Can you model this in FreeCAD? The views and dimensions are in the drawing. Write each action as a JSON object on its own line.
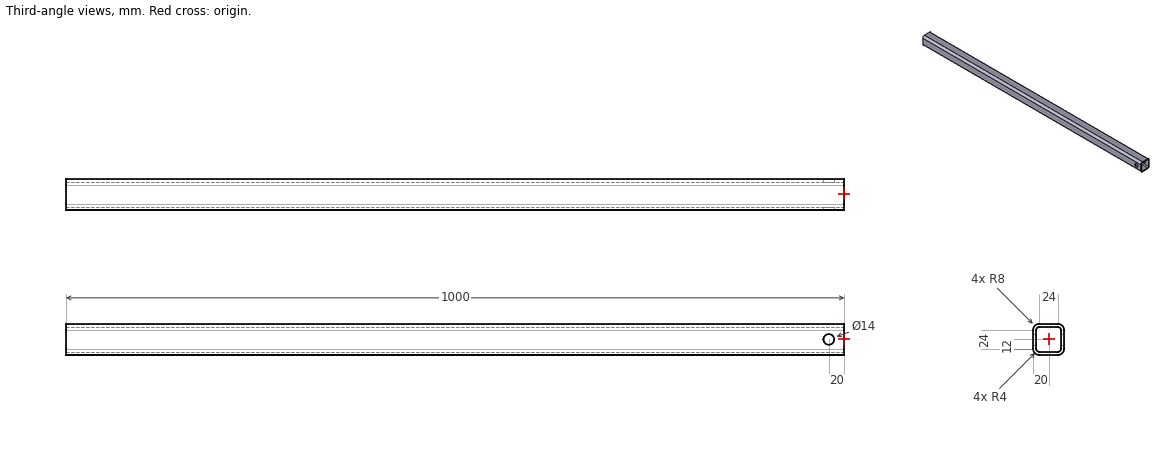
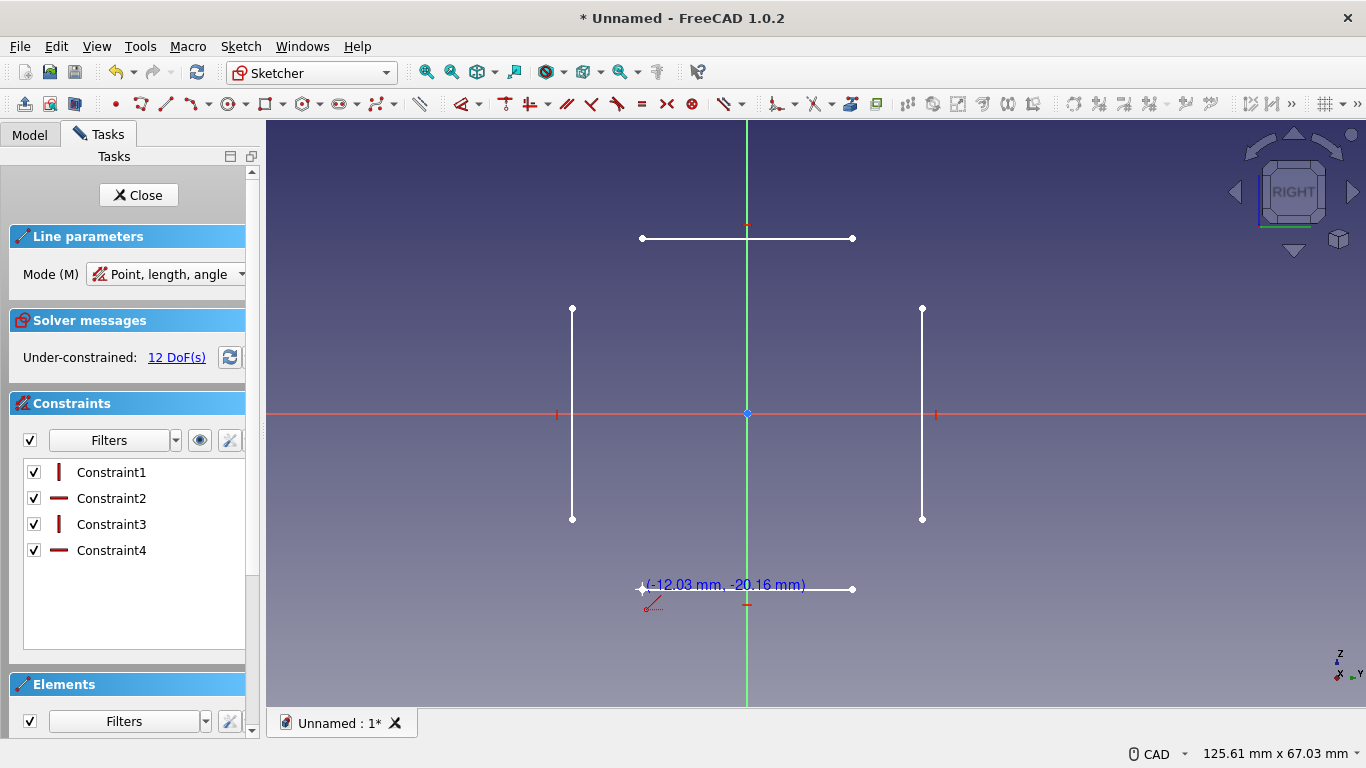
{"action": "left_click", "coordinate": [190, 104]}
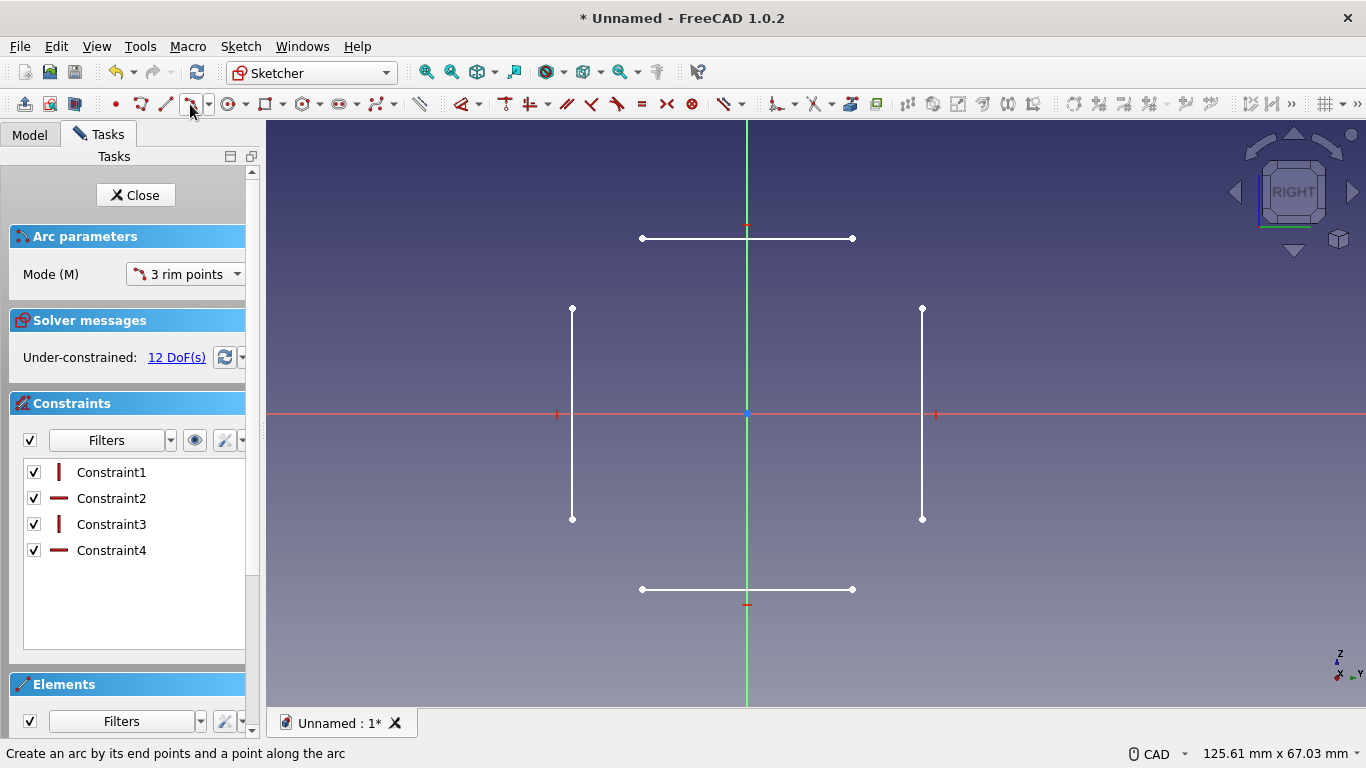
{"action": "left_click", "coordinate": [572, 309]}
{"action": "left_click", "coordinate": [642, 239]}
{"action": "left_click", "coordinate": [593, 259]}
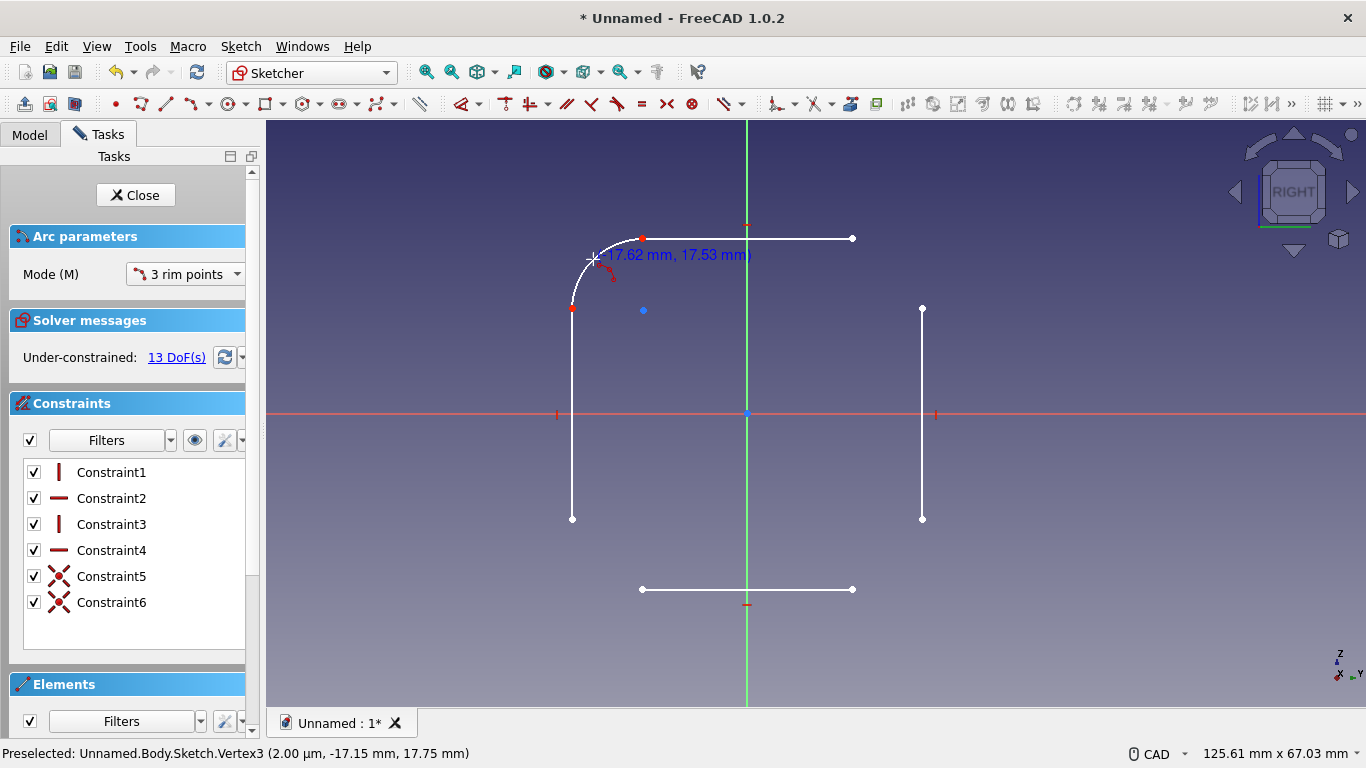
{"action": "left_click", "coordinate": [852, 239]}
{"action": "left_click", "coordinate": [922, 309]}
{"action": "left_click", "coordinate": [902, 259]}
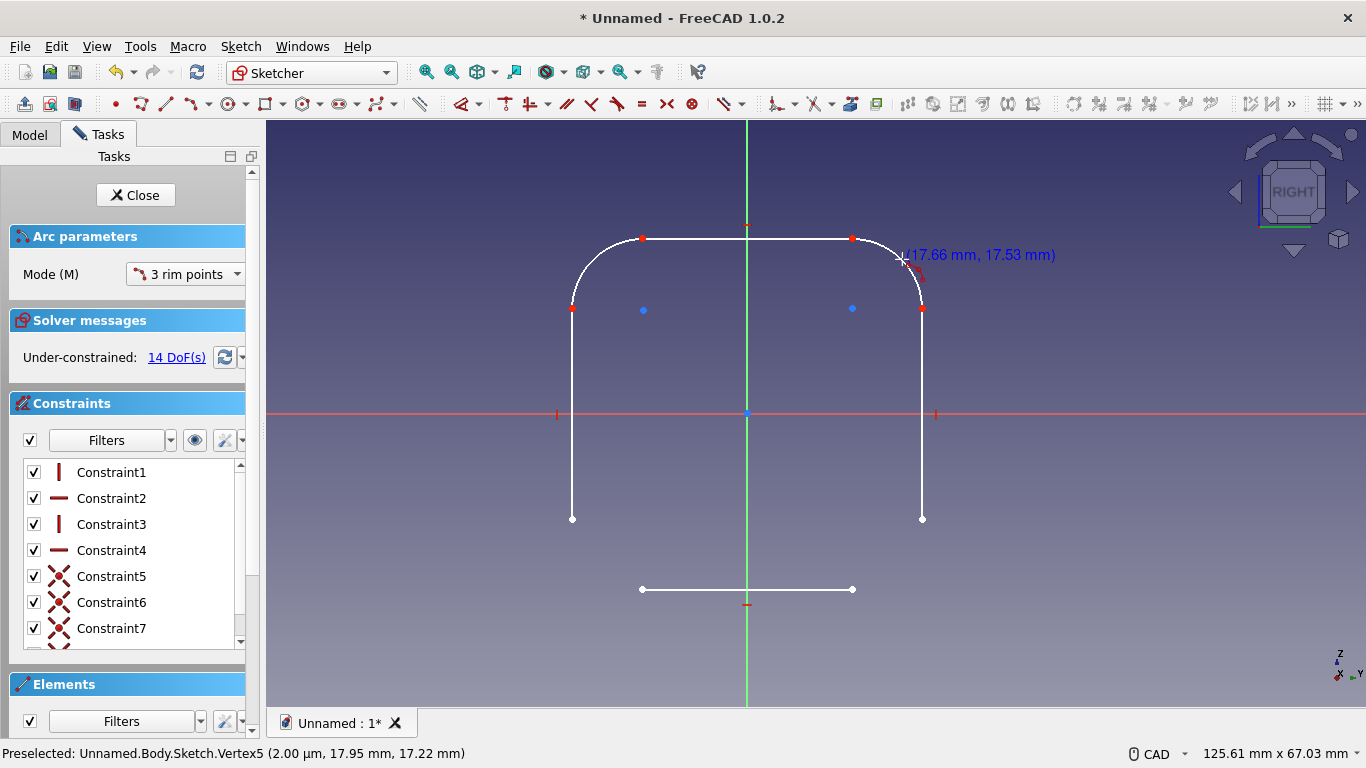
{"action": "left_click", "coordinate": [922, 520]}
{"action": "left_click", "coordinate": [852, 590]}
{"action": "left_click", "coordinate": [902, 568]}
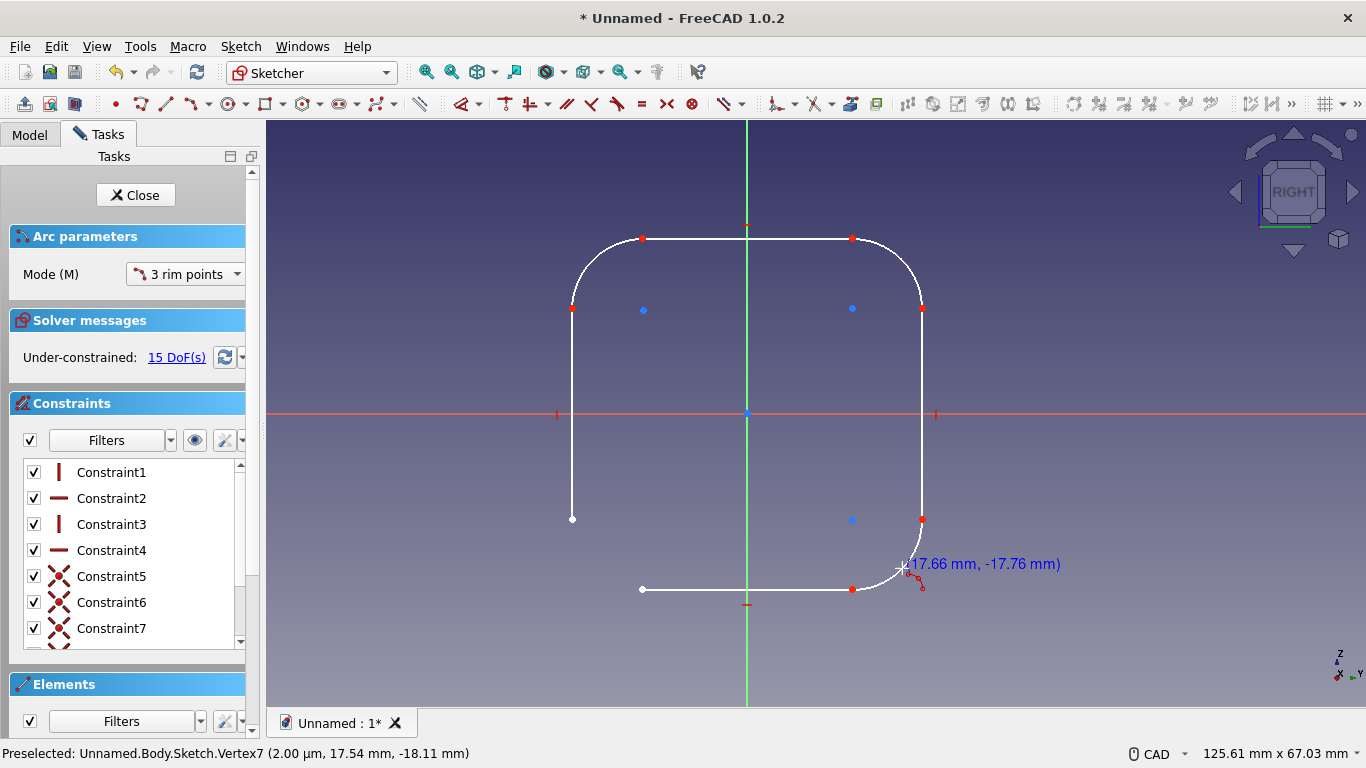
{"action": "left_click", "coordinate": [642, 590]}
{"action": "left_click", "coordinate": [572, 520]}
{"action": "left_click", "coordinate": [593, 568]}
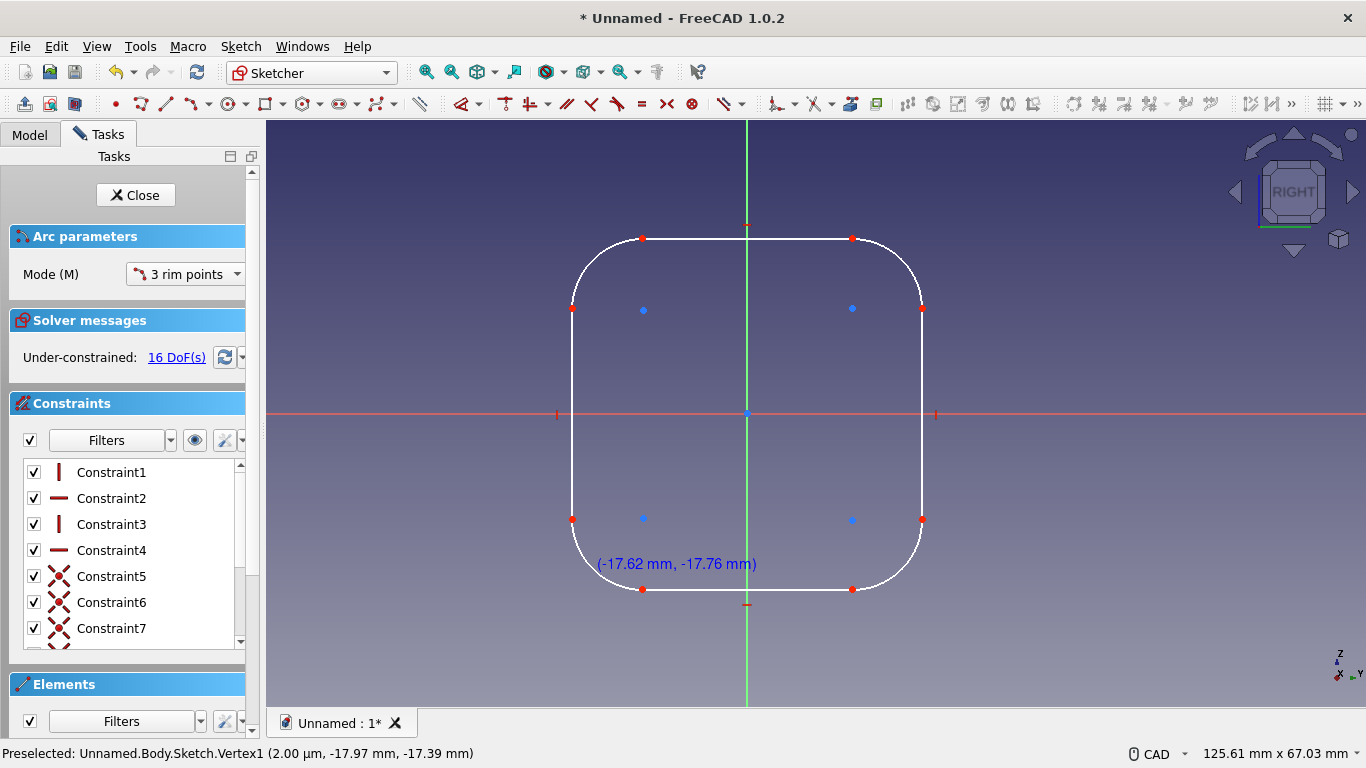
{"action": "left_click", "coordinate": [166, 104]}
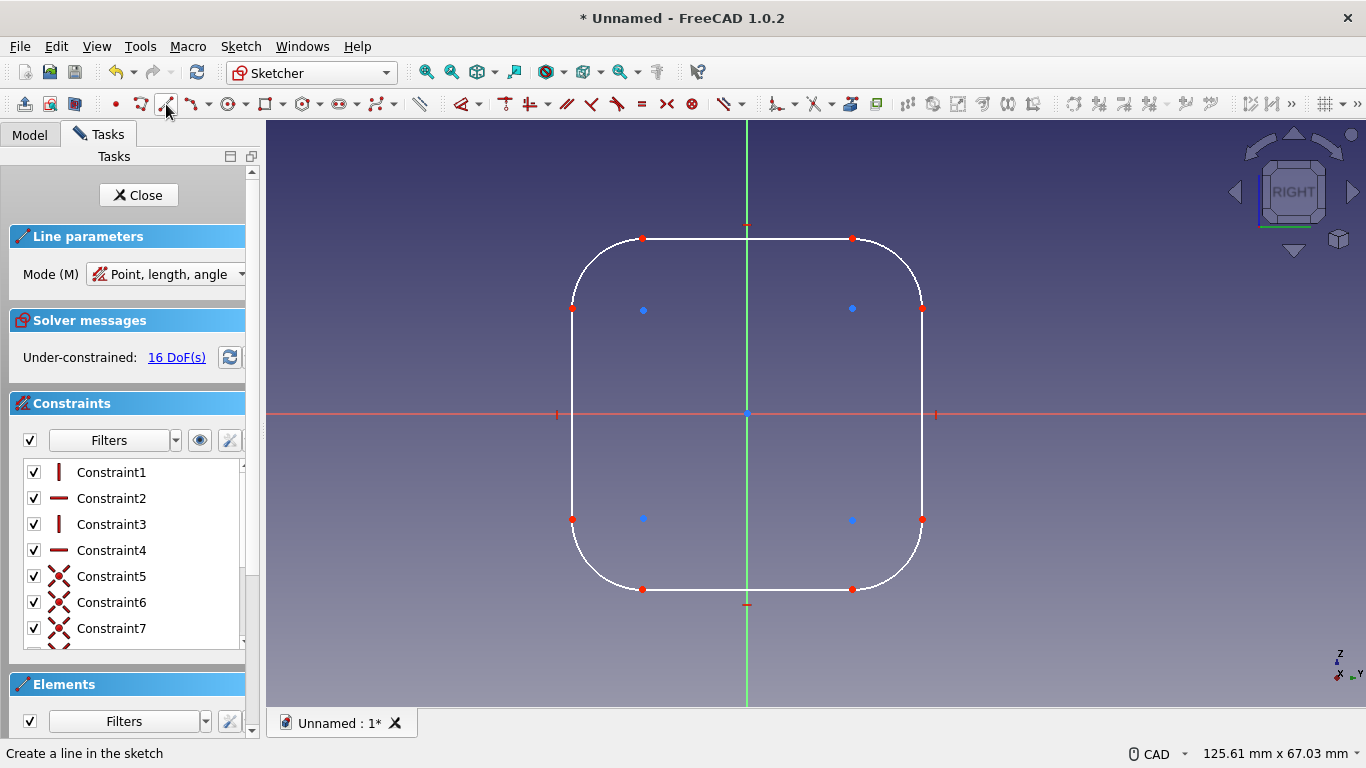
{"action": "left_click", "coordinate": [607, 308]}
{"action": "left_click", "coordinate": [607, 519]}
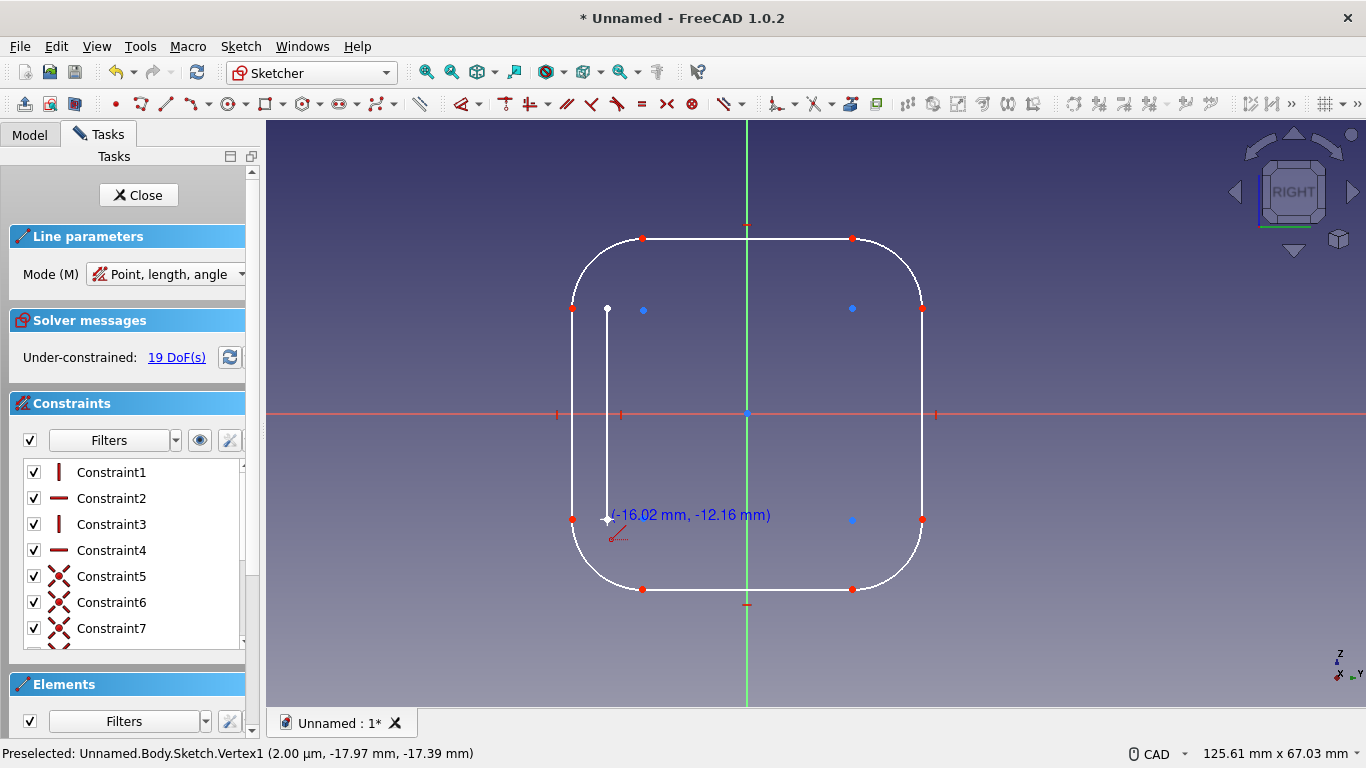
{"action": "left_click", "coordinate": [642, 554]}
{"action": "left_click", "coordinate": [852, 554]}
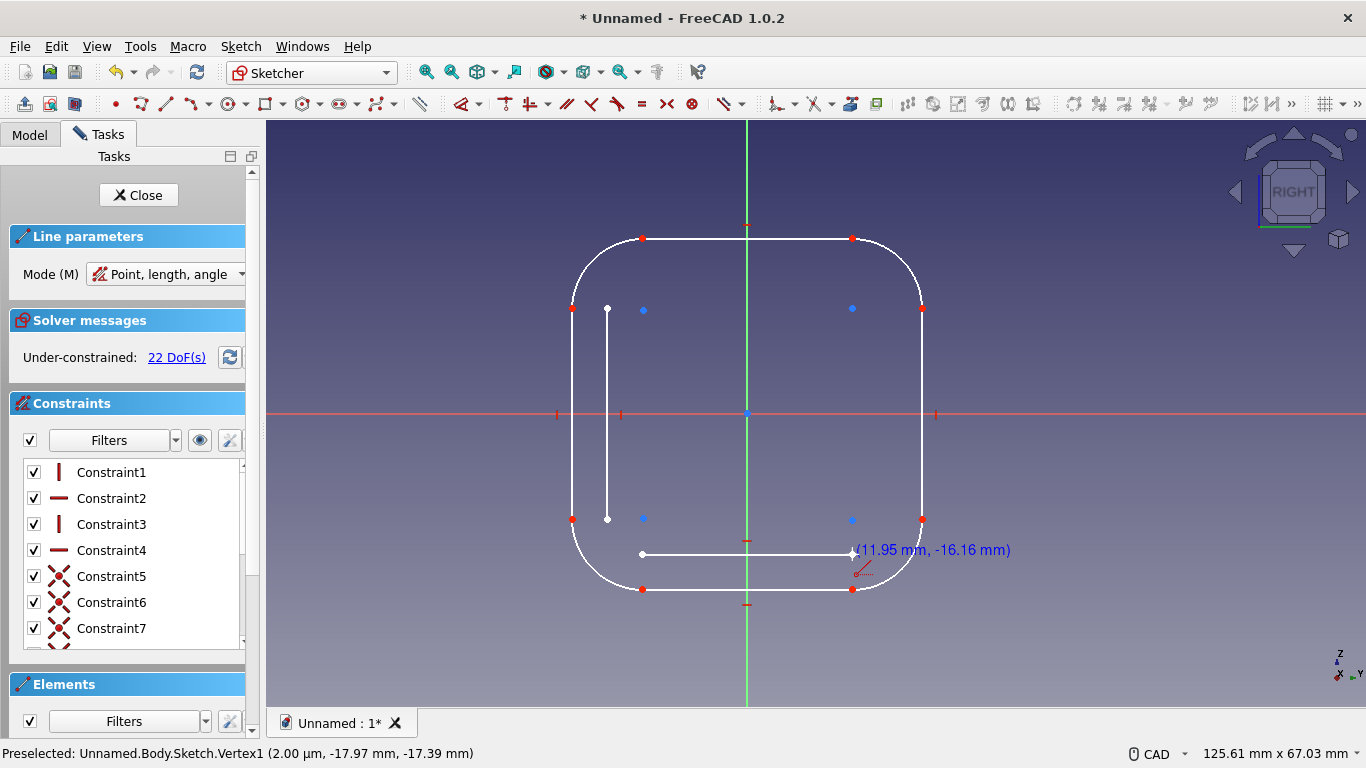
{"action": "left_click", "coordinate": [887, 519]}
{"action": "left_click", "coordinate": [887, 308]}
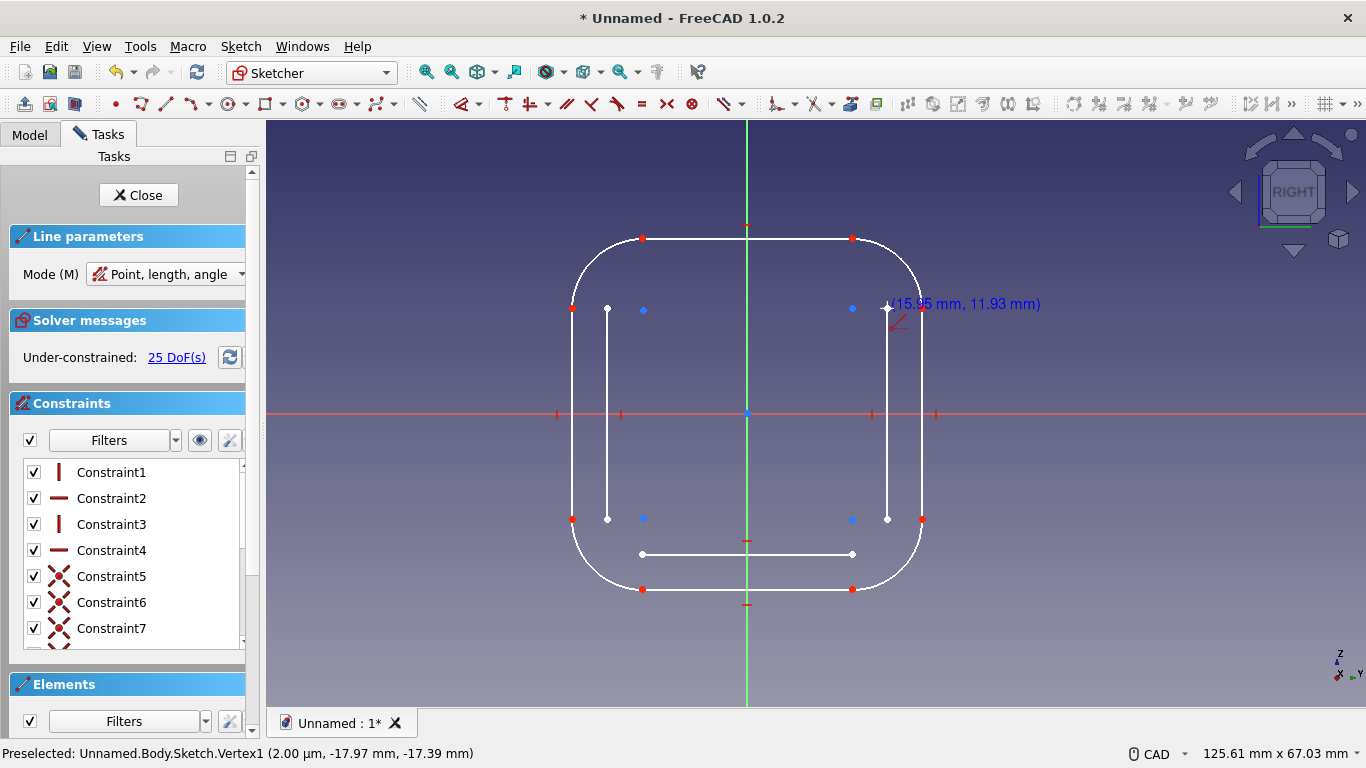
{"action": "left_click", "coordinate": [852, 273]}
{"action": "left_click", "coordinate": [642, 273]}